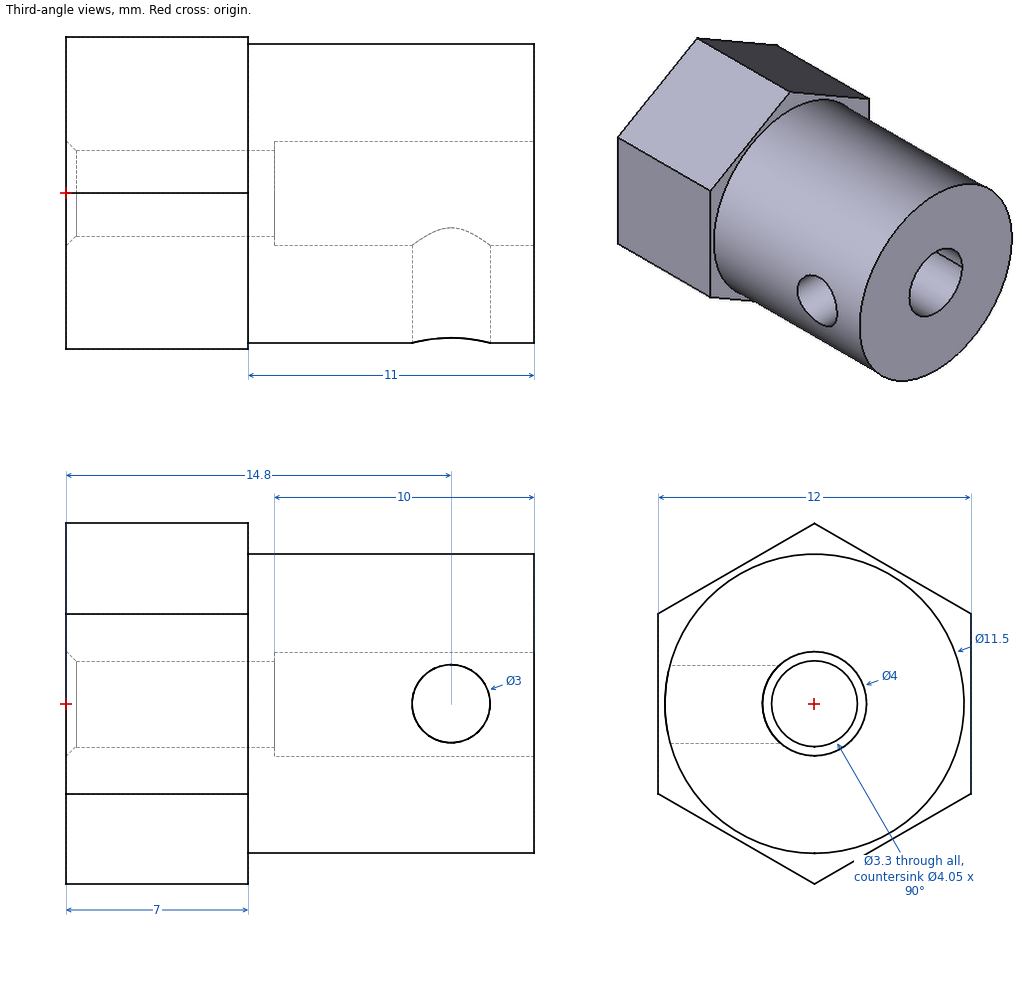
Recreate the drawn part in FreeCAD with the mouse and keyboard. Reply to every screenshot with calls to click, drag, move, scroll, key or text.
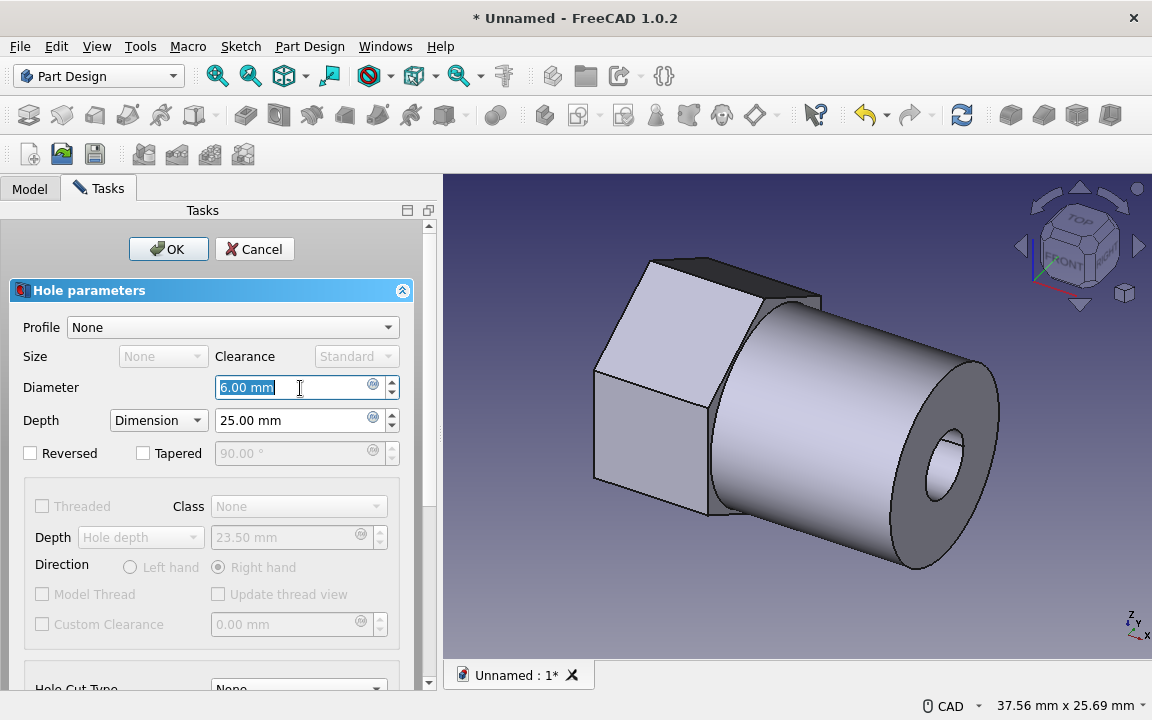
text(3.3)
key(Tab)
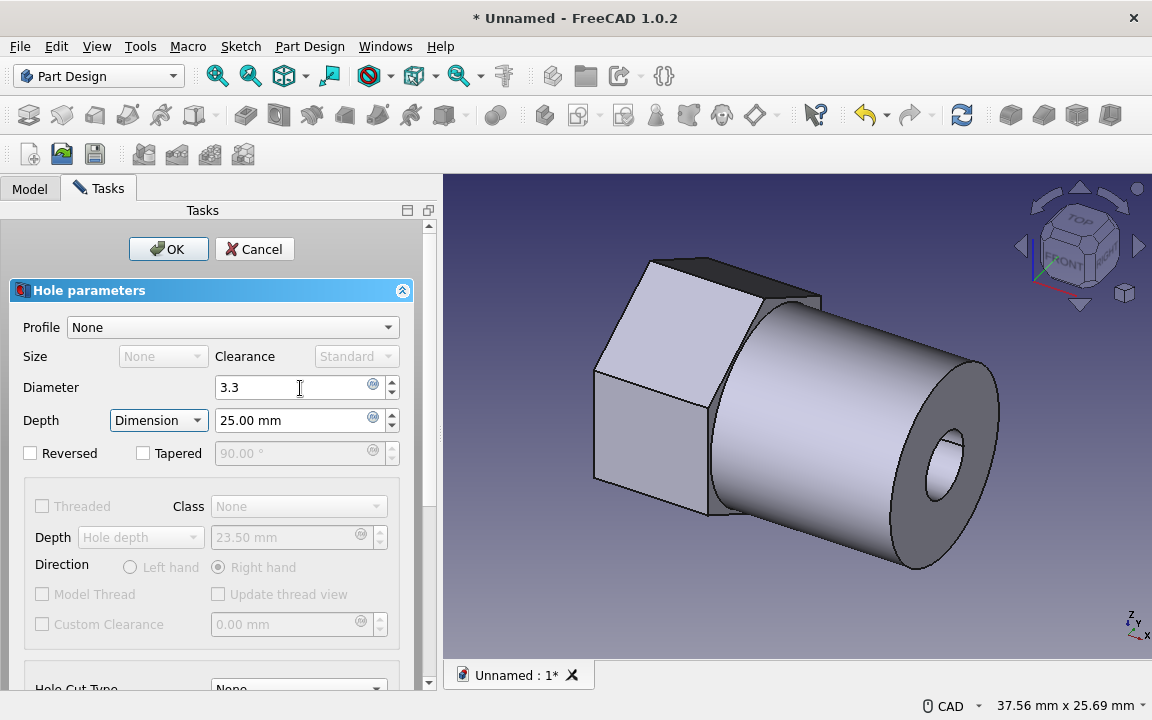
click(160, 420)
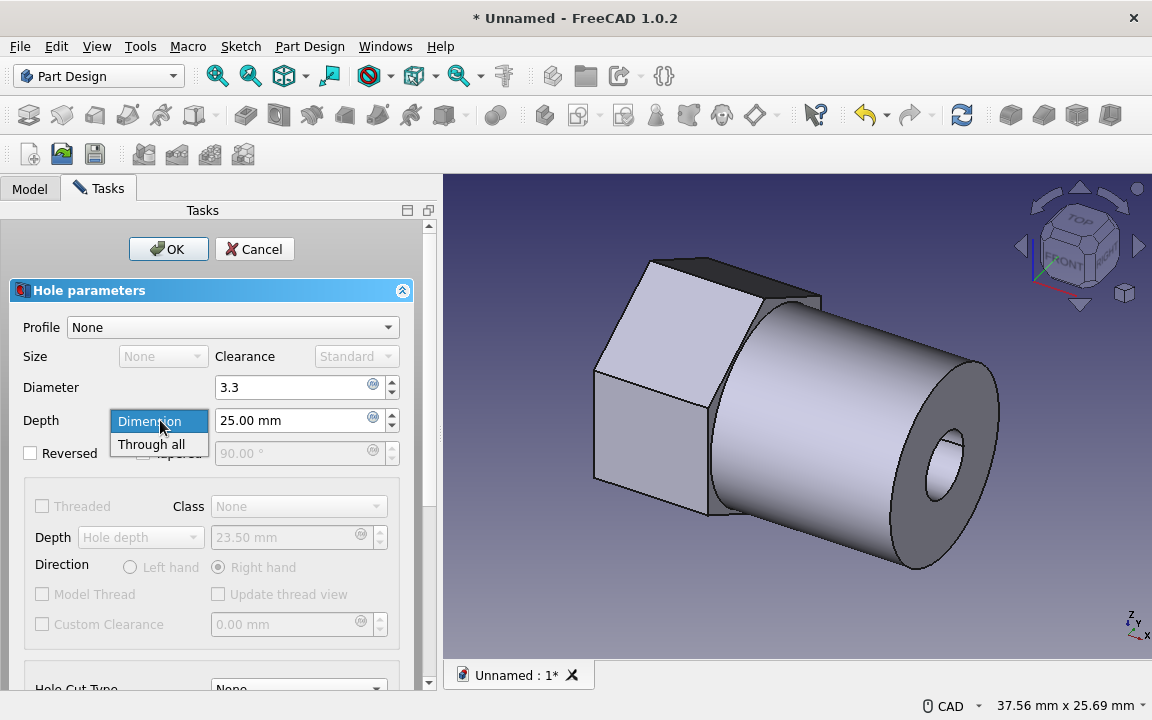
click(158, 444)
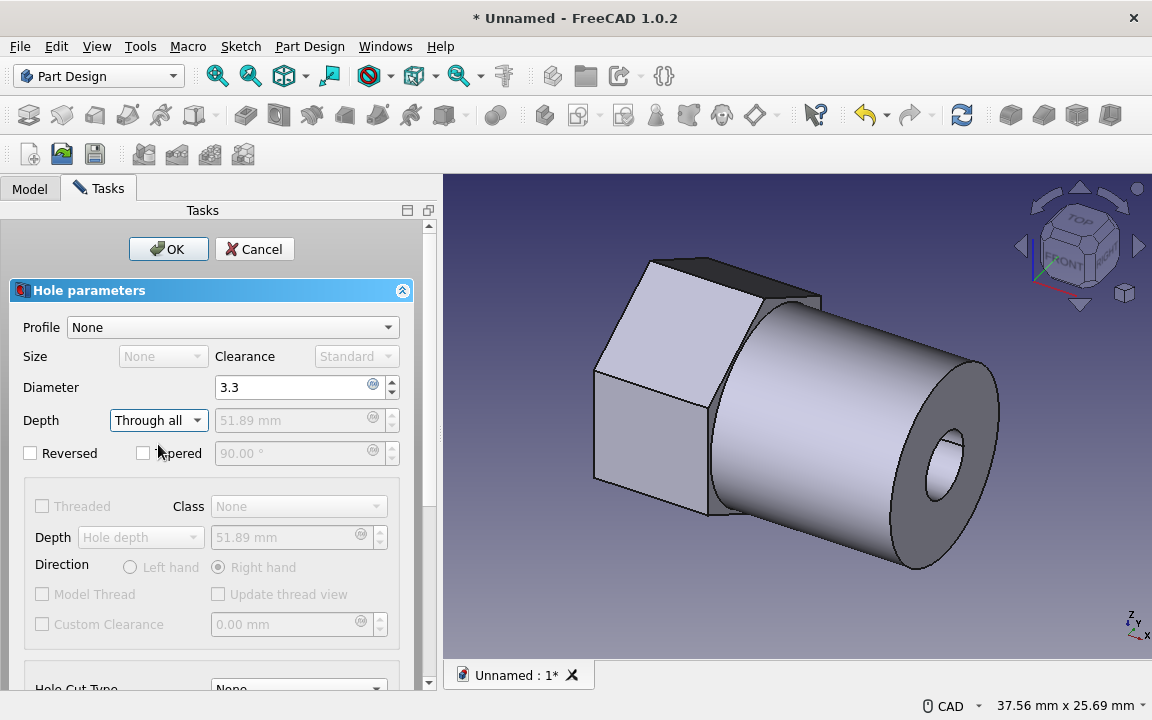
click(31, 453)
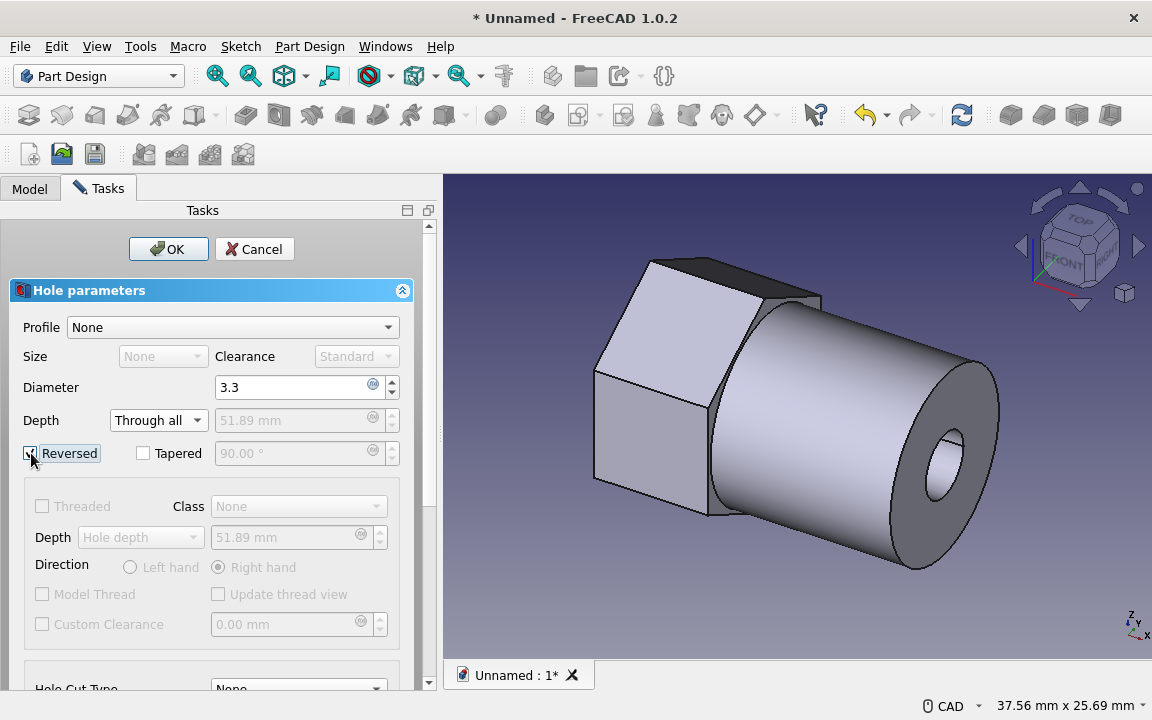
scroll(429, 455, down, 2)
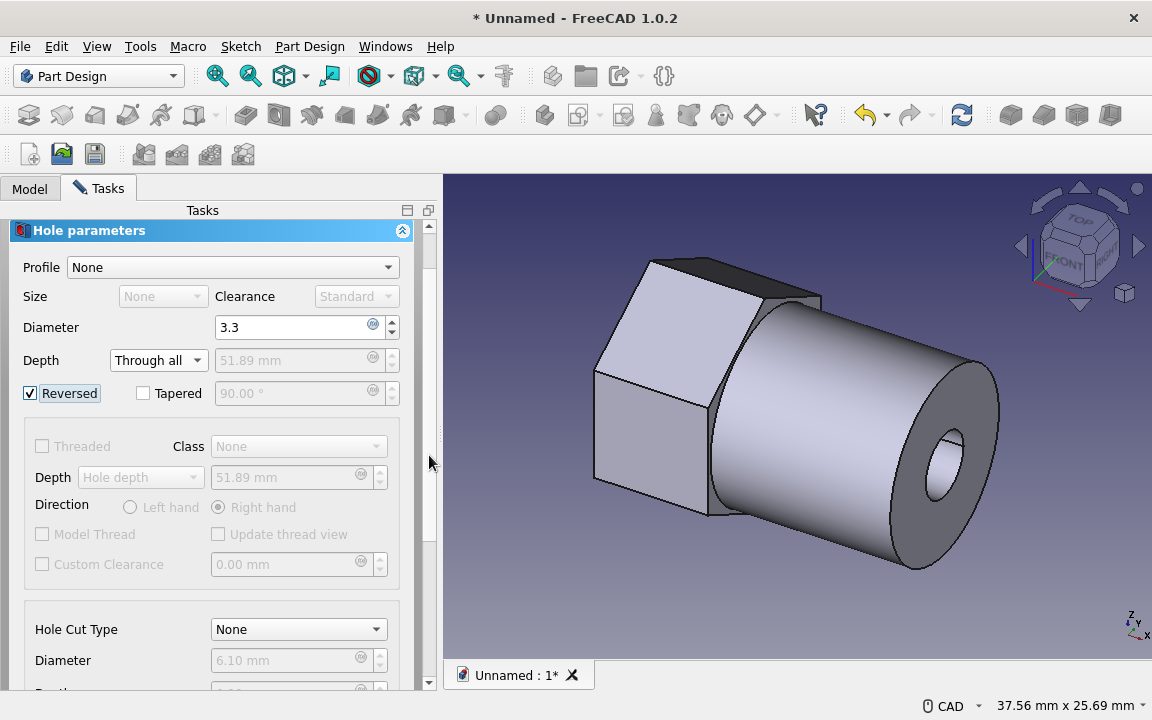
click(300, 570)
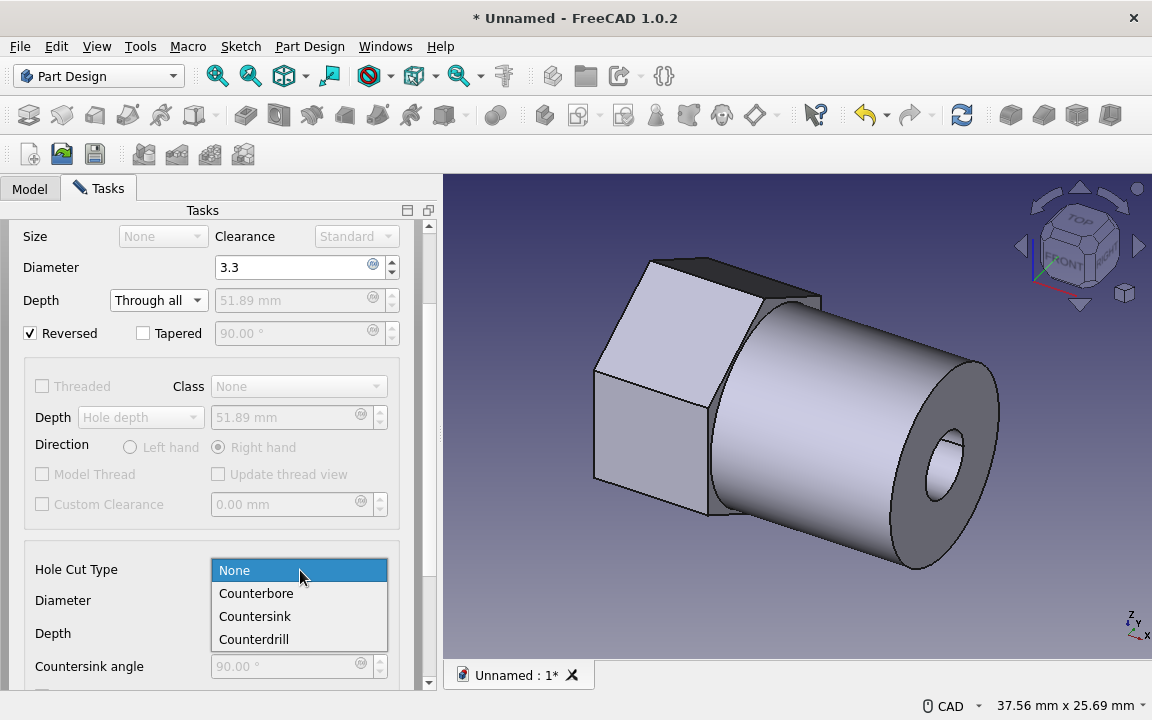
click(298, 616)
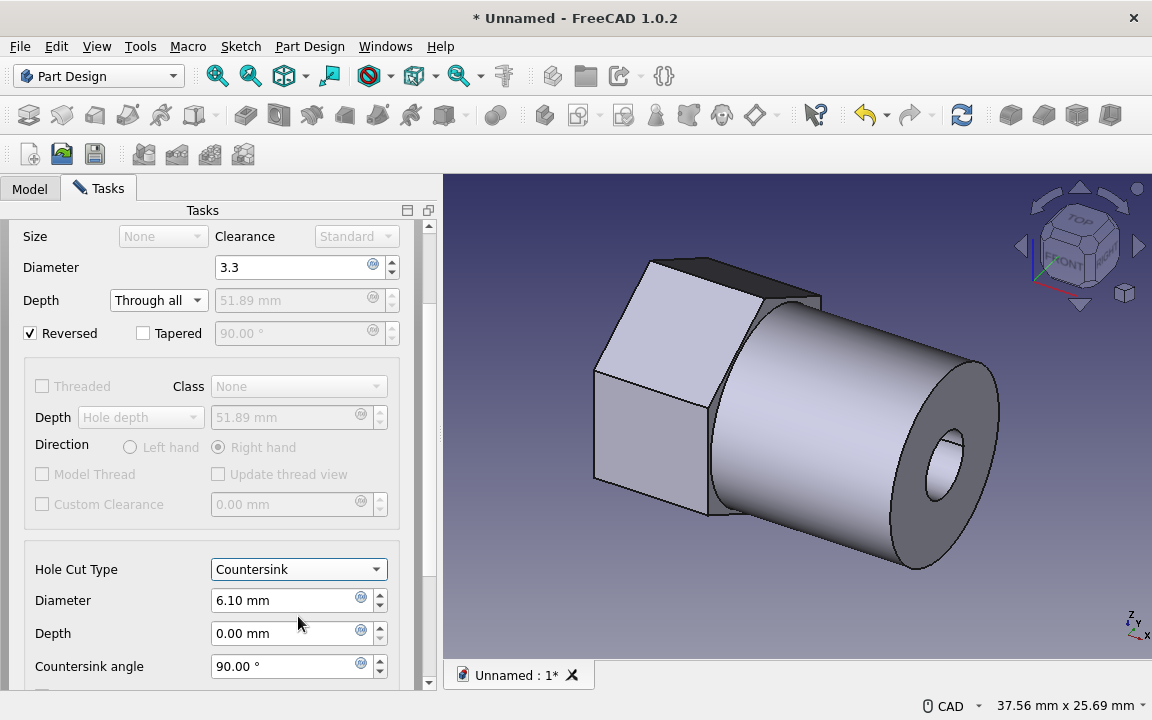
triple_click(292, 600)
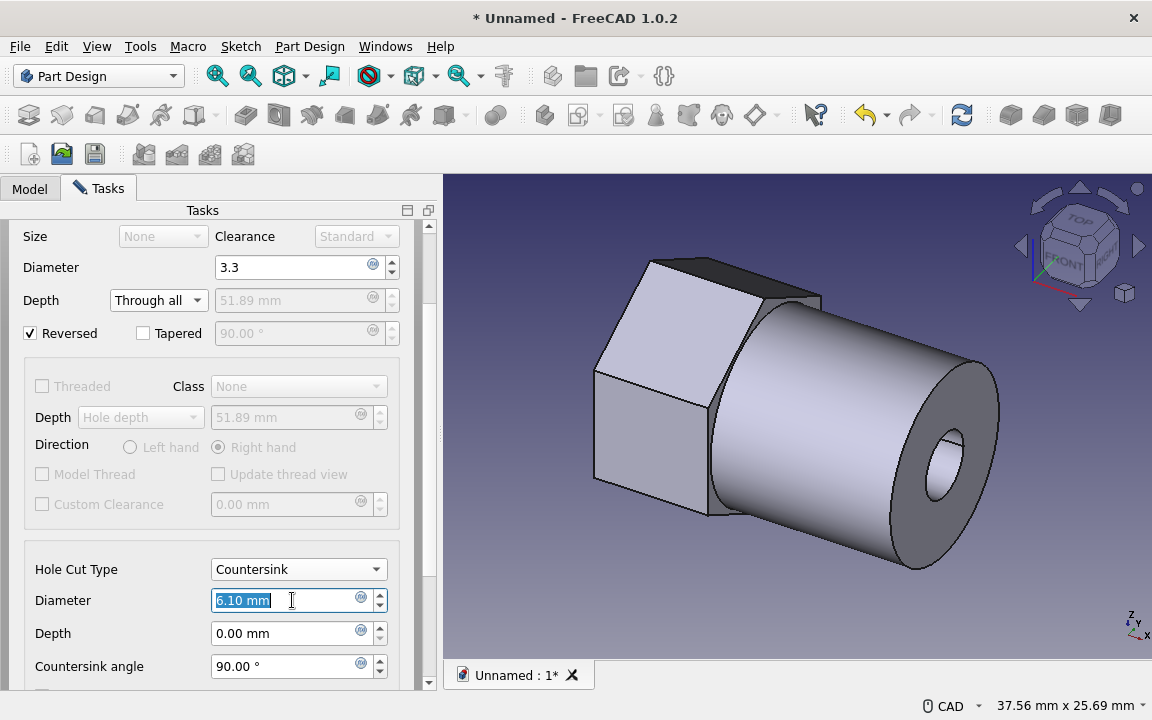
text(4.05)
key(Tab)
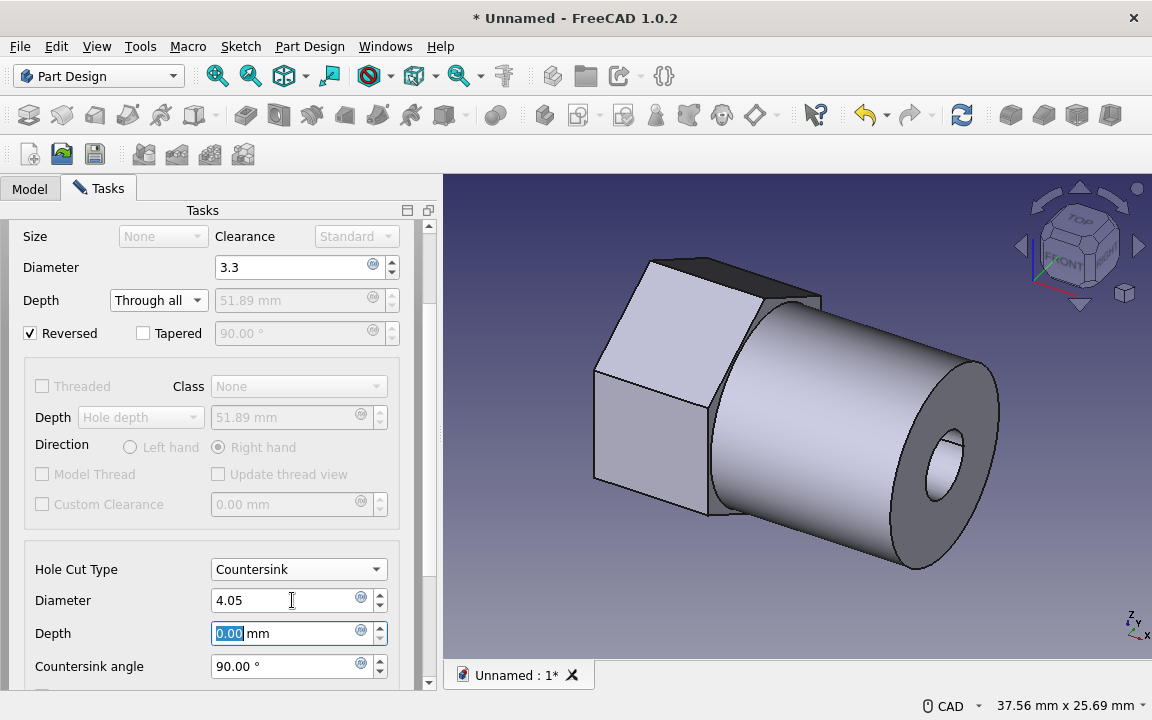
scroll(429, 455, up, 3)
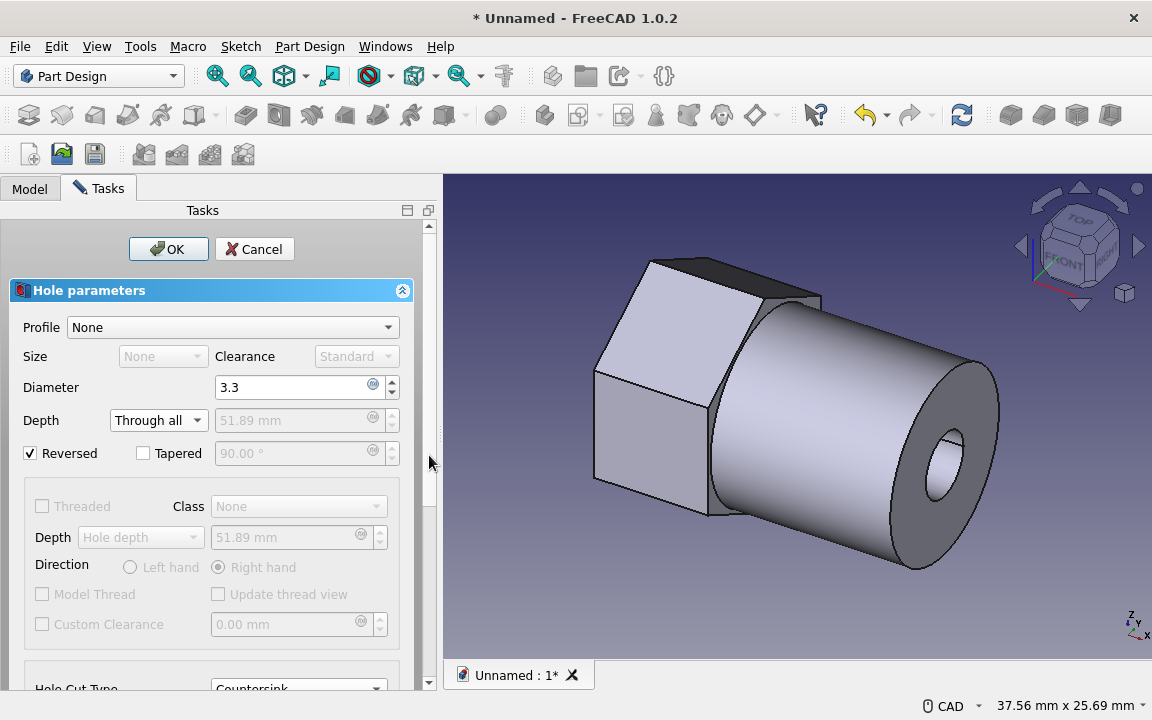
click(169, 249)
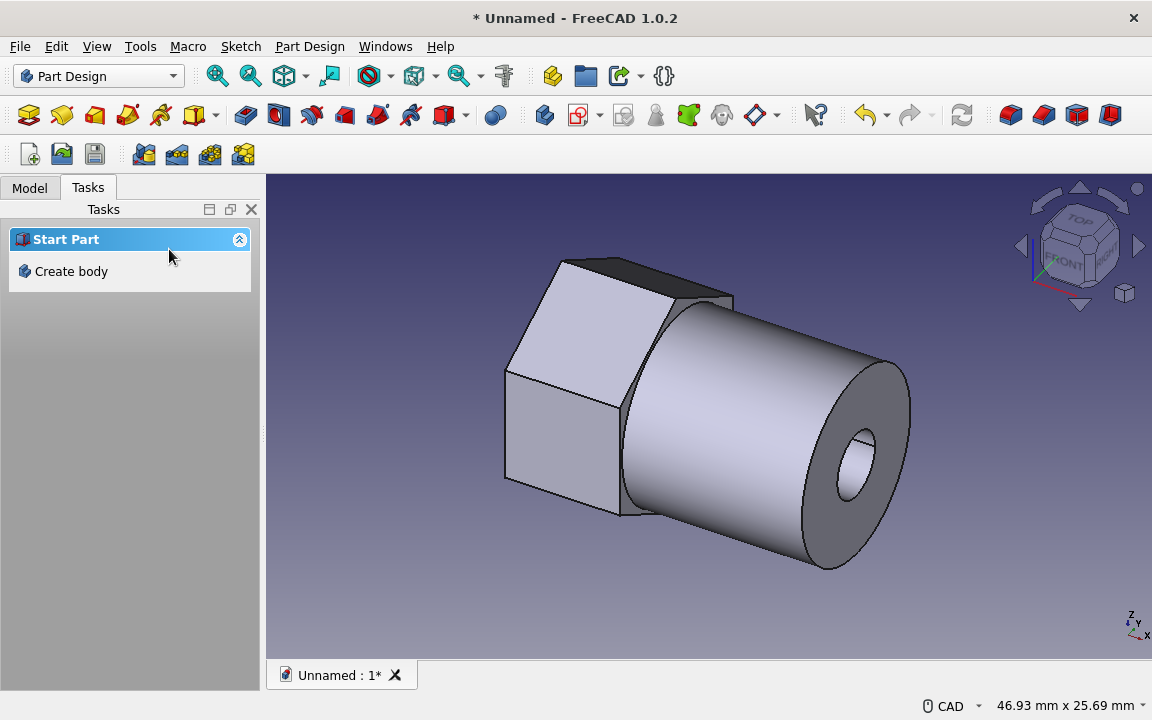
click(578, 116)